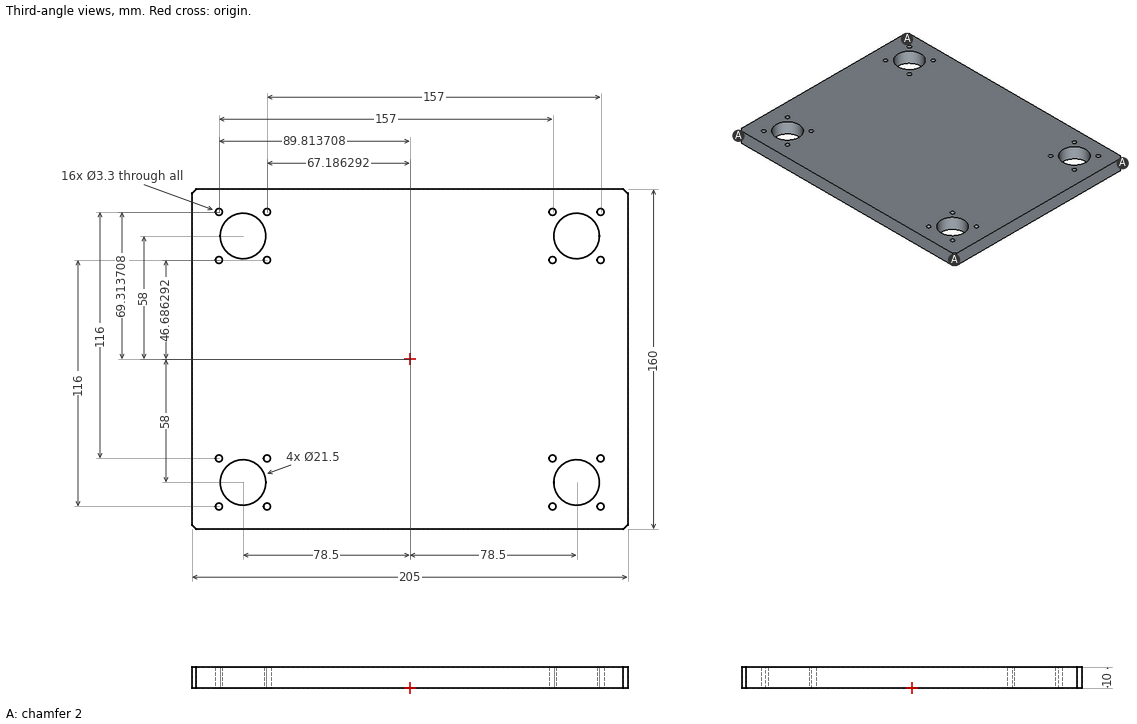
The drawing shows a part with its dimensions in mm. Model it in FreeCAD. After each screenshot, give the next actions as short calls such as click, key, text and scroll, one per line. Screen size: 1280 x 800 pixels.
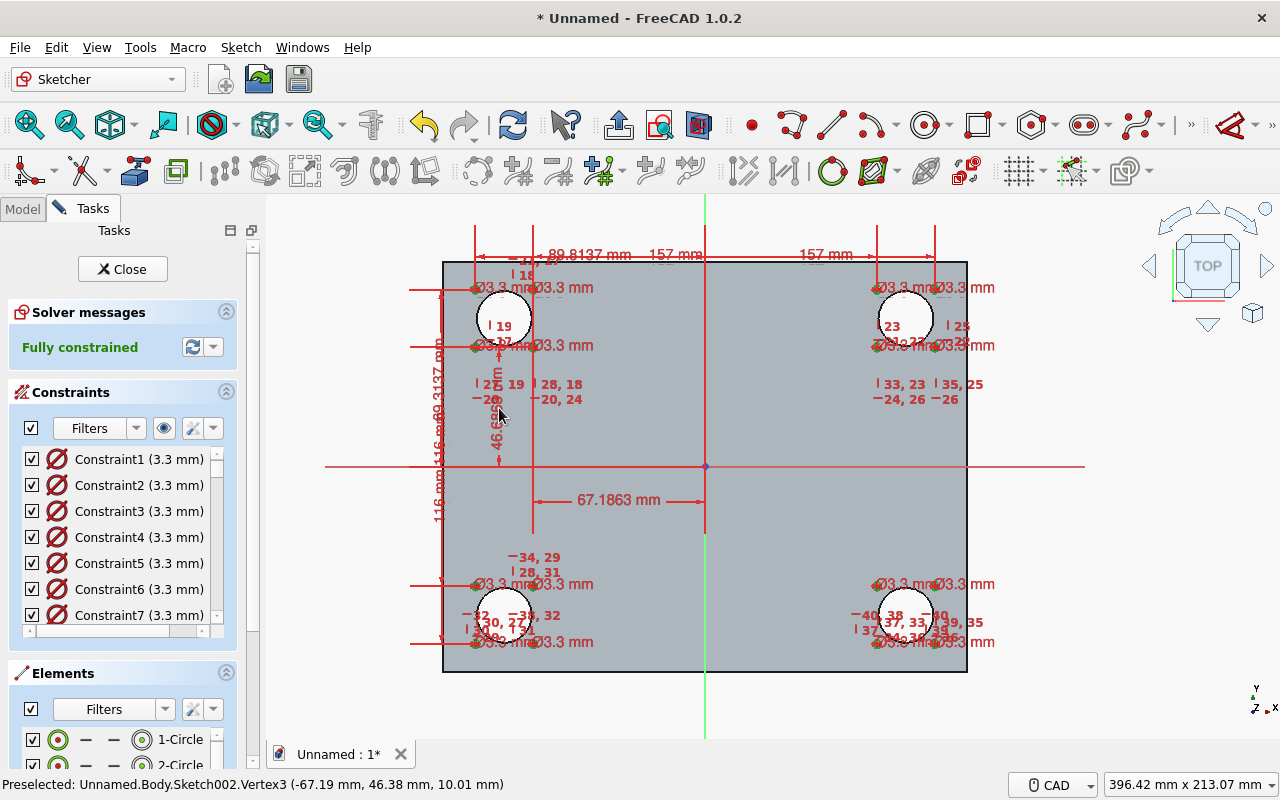
click(123, 269)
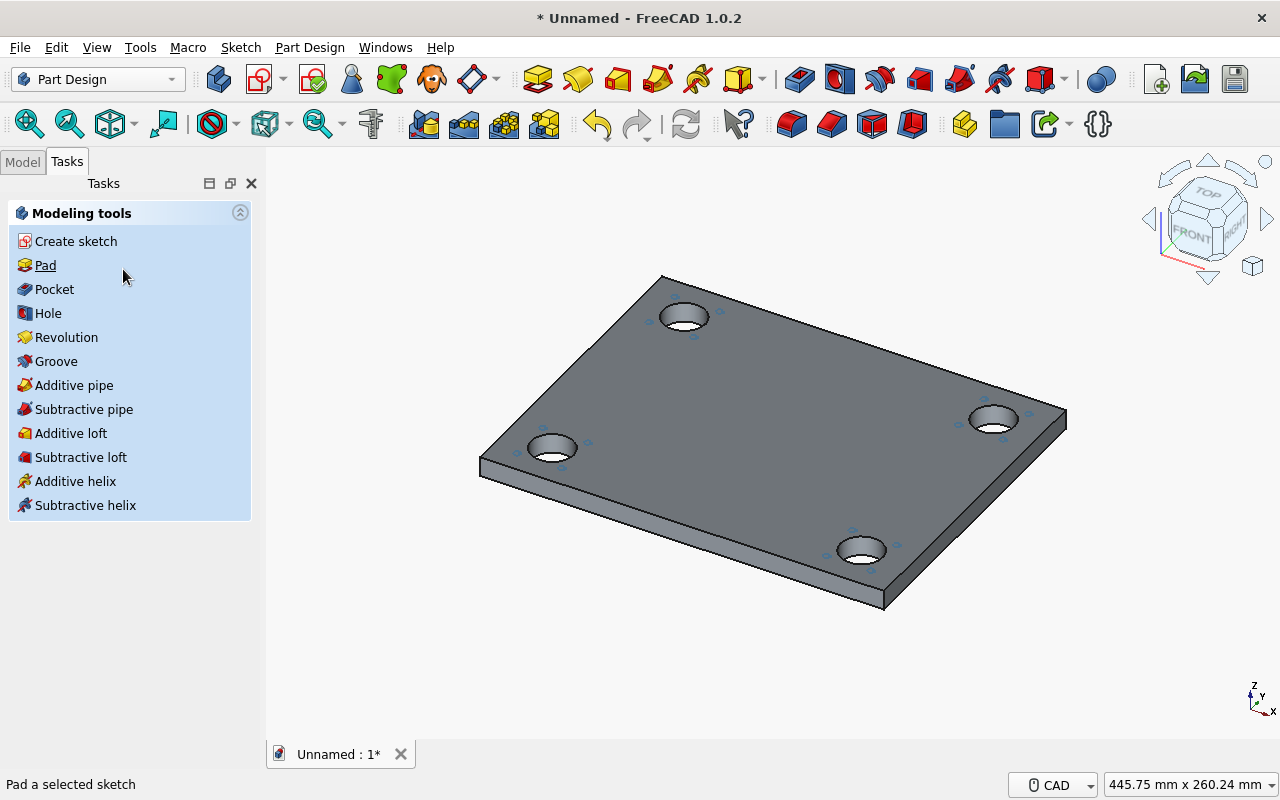
click(840, 80)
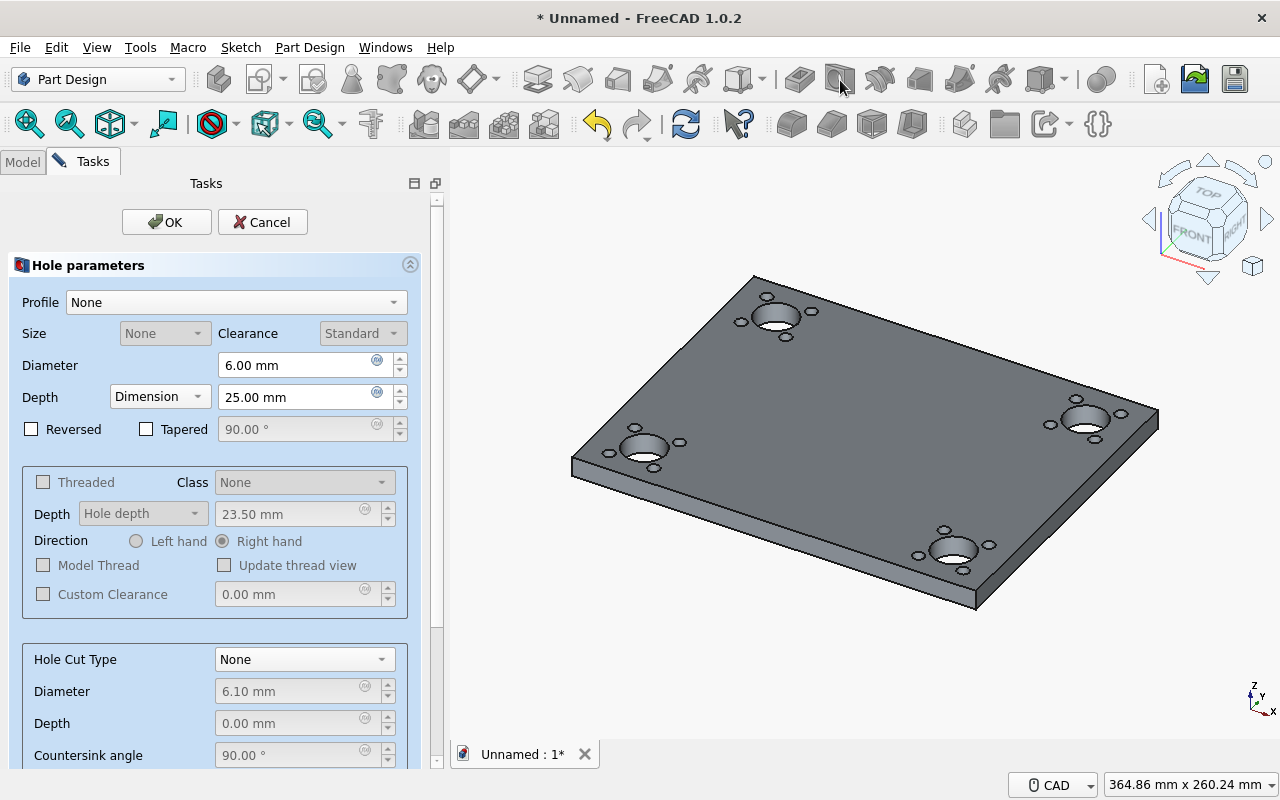
triple_click(305, 365)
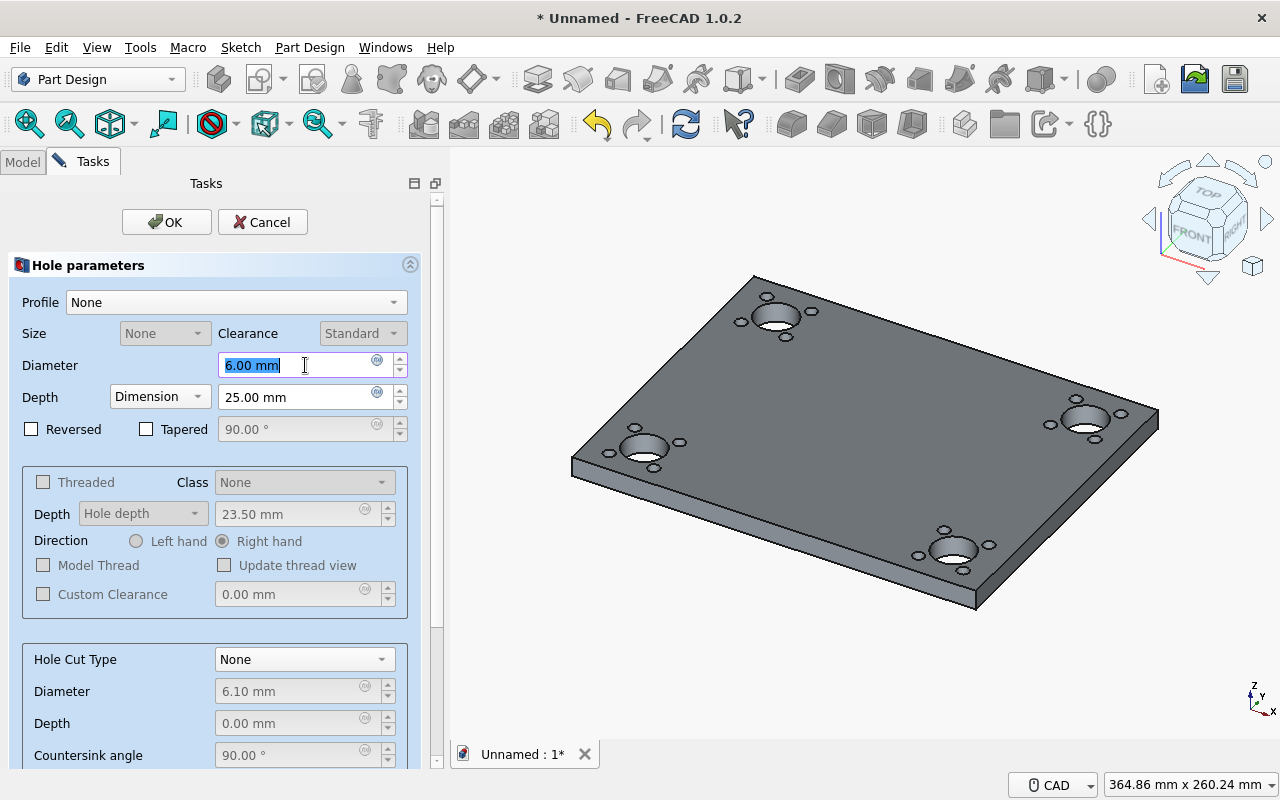
text(3.3)
key(Tab)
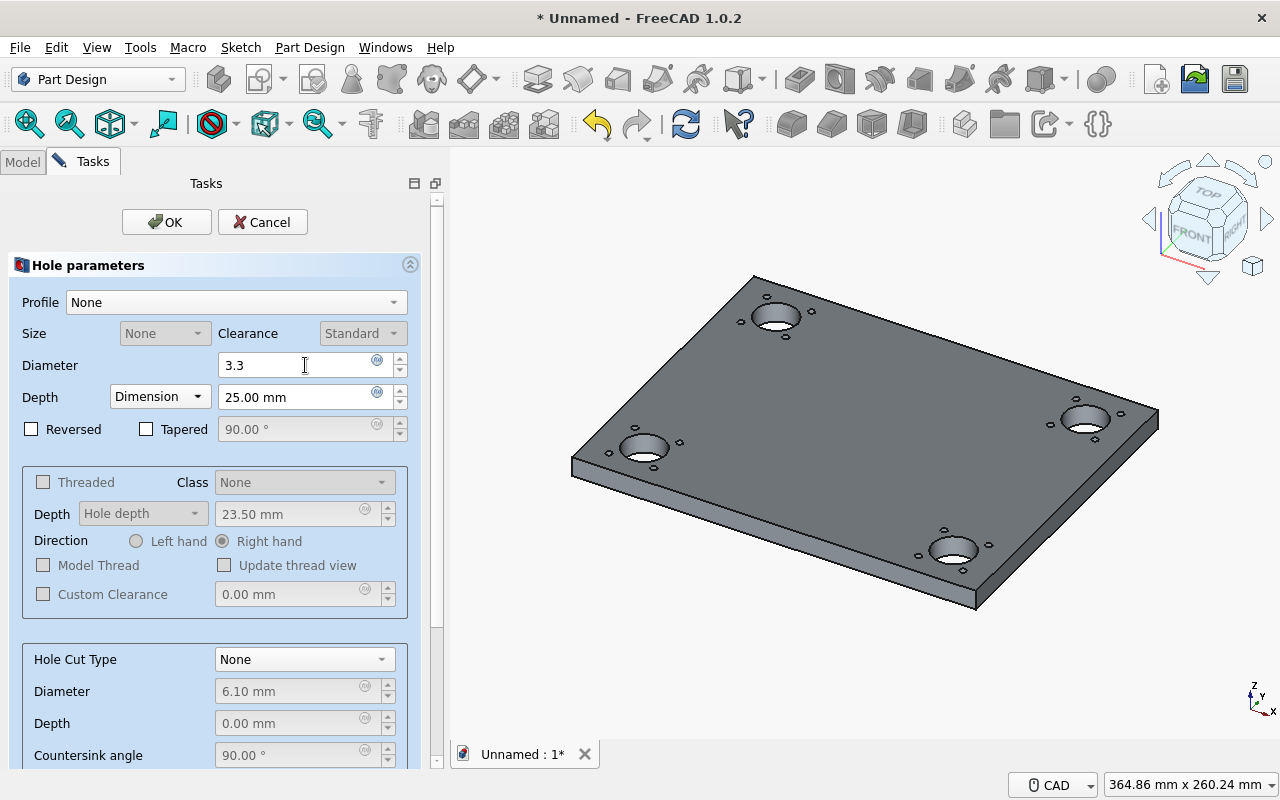
click(161, 396)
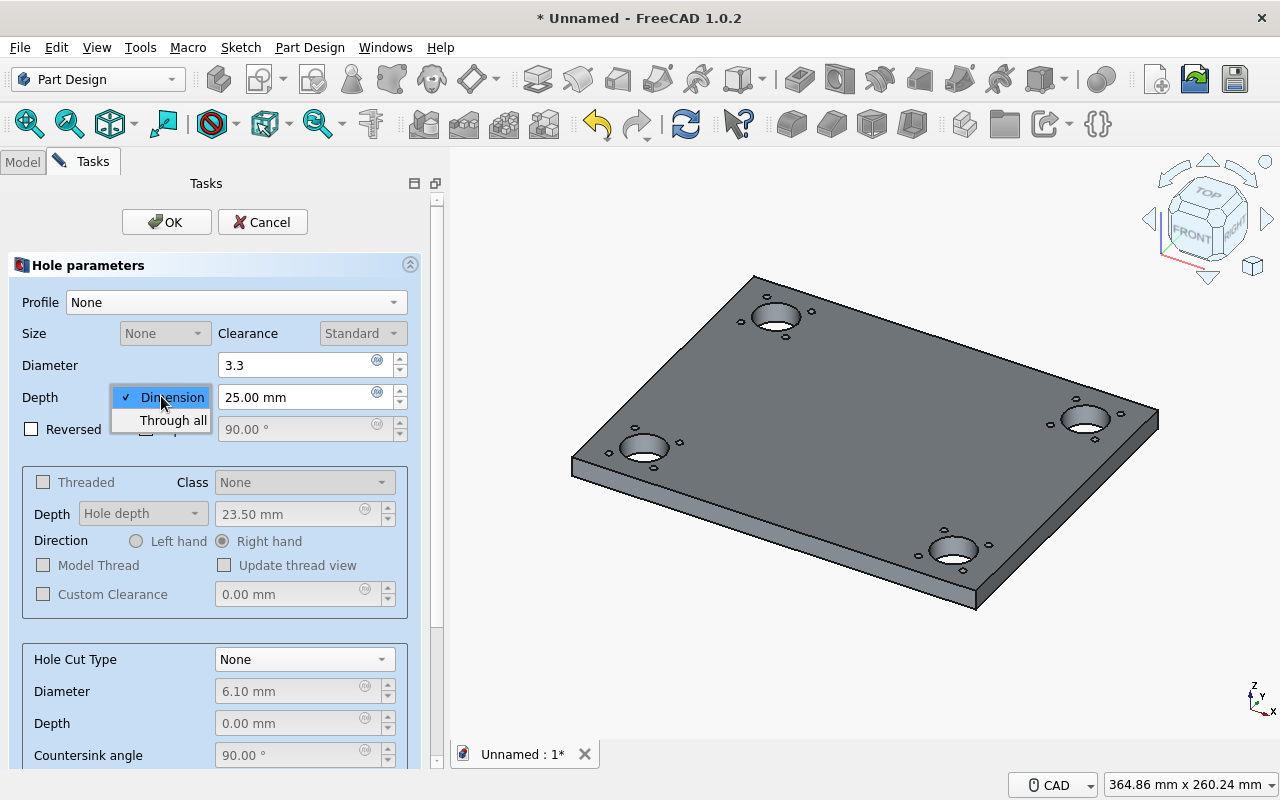
click(160, 420)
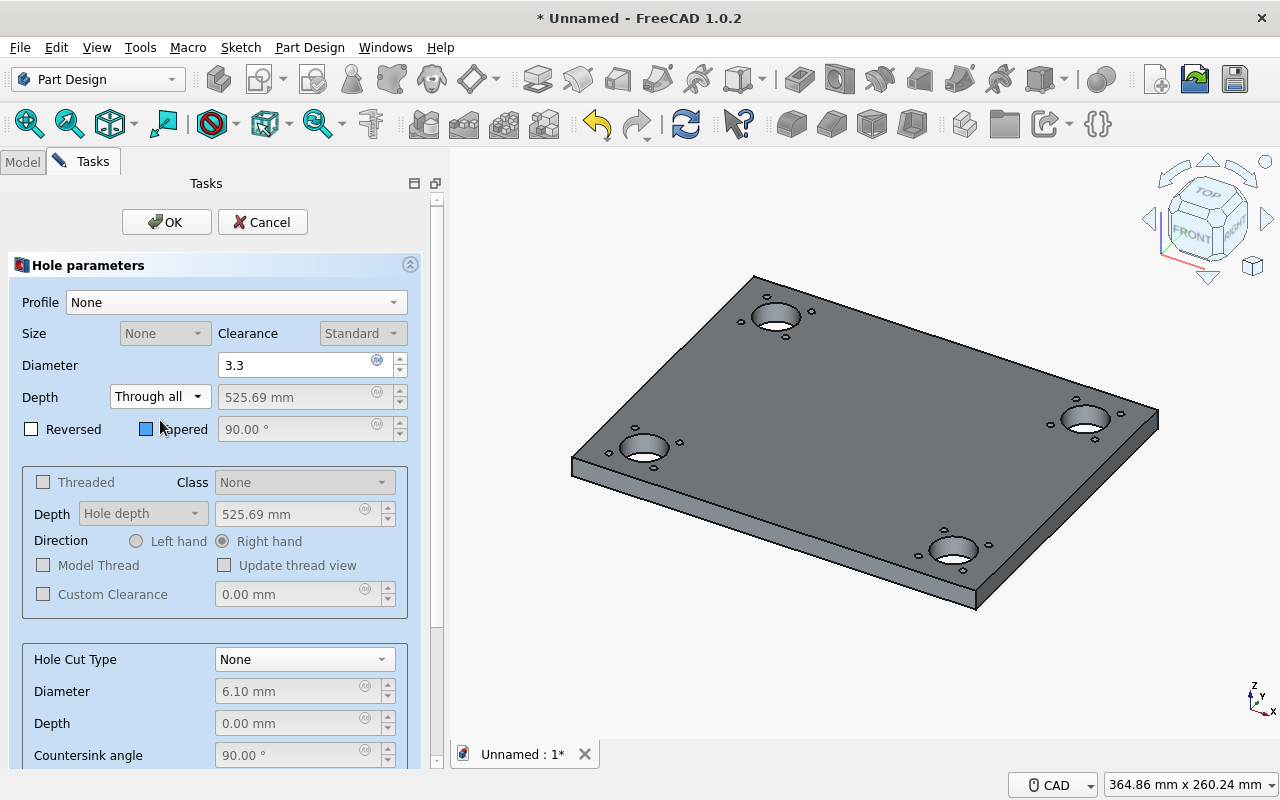
click(167, 222)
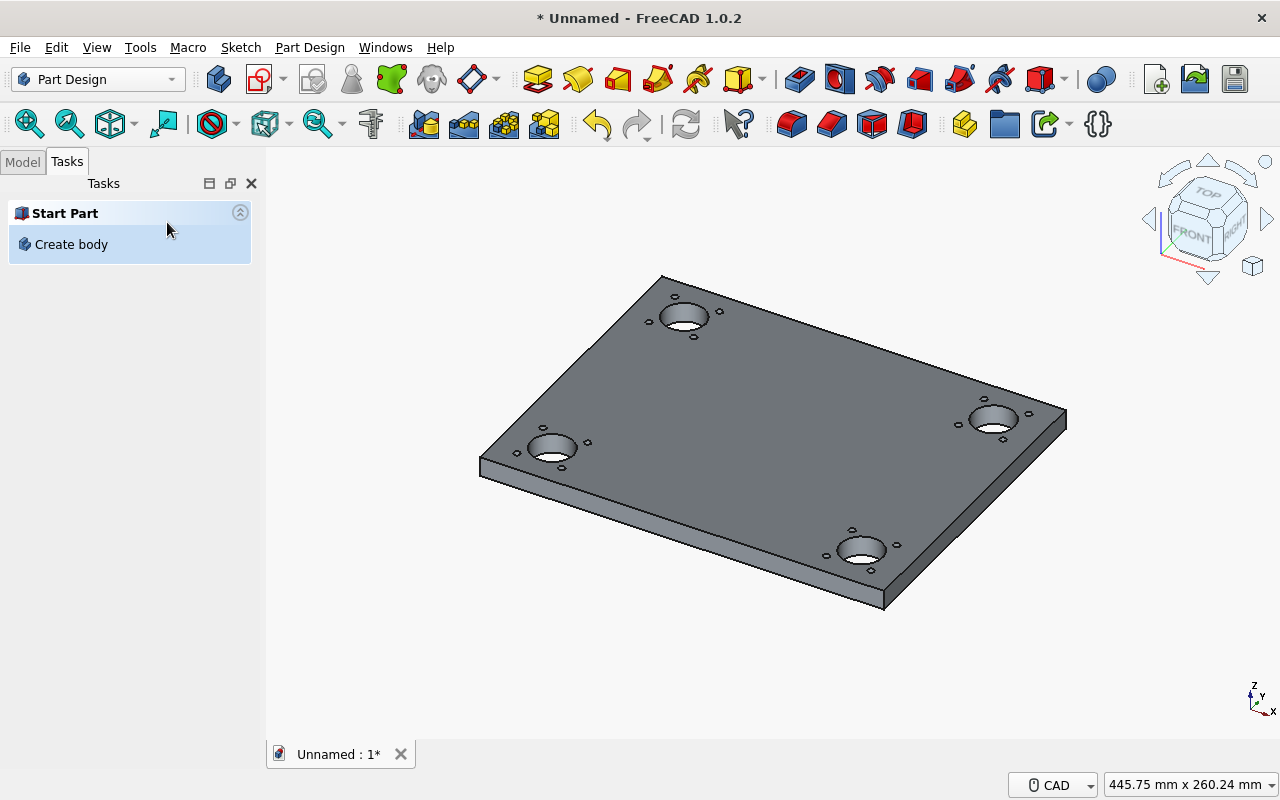
click(884, 599)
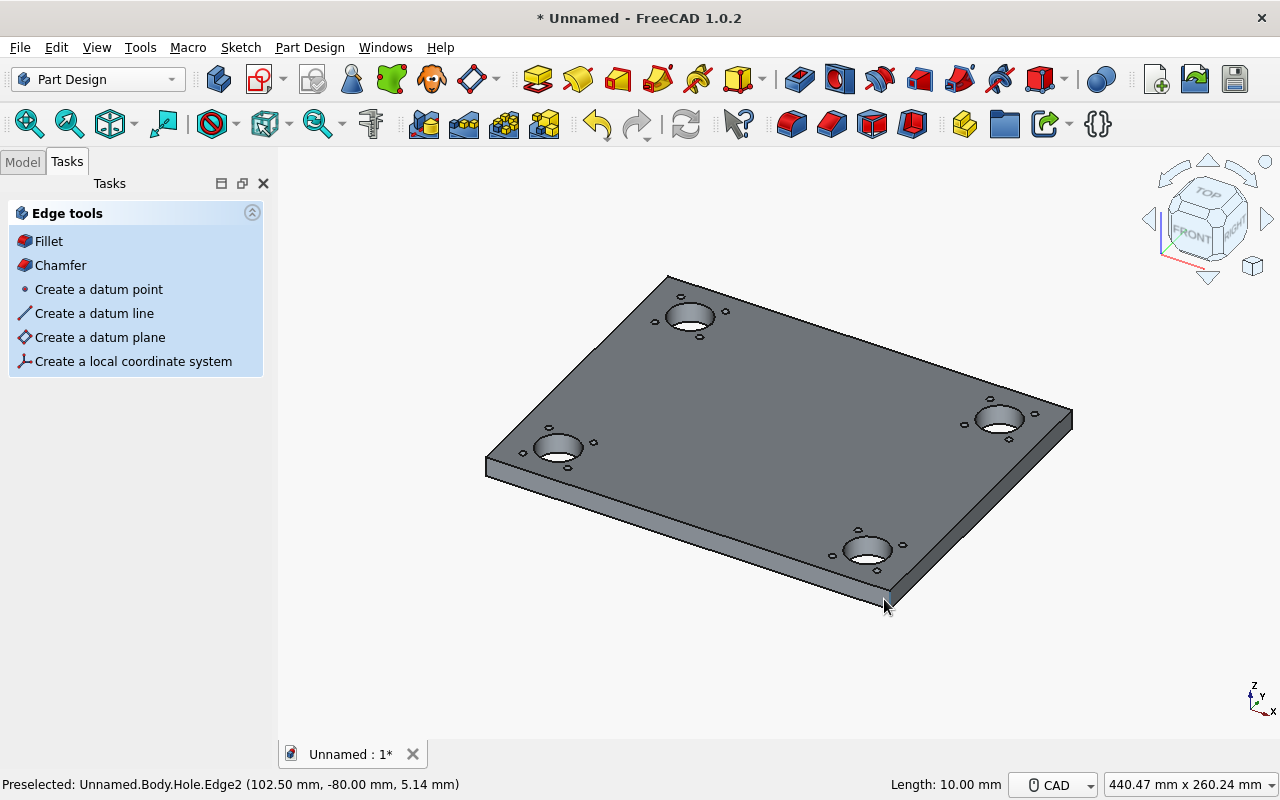
key(0)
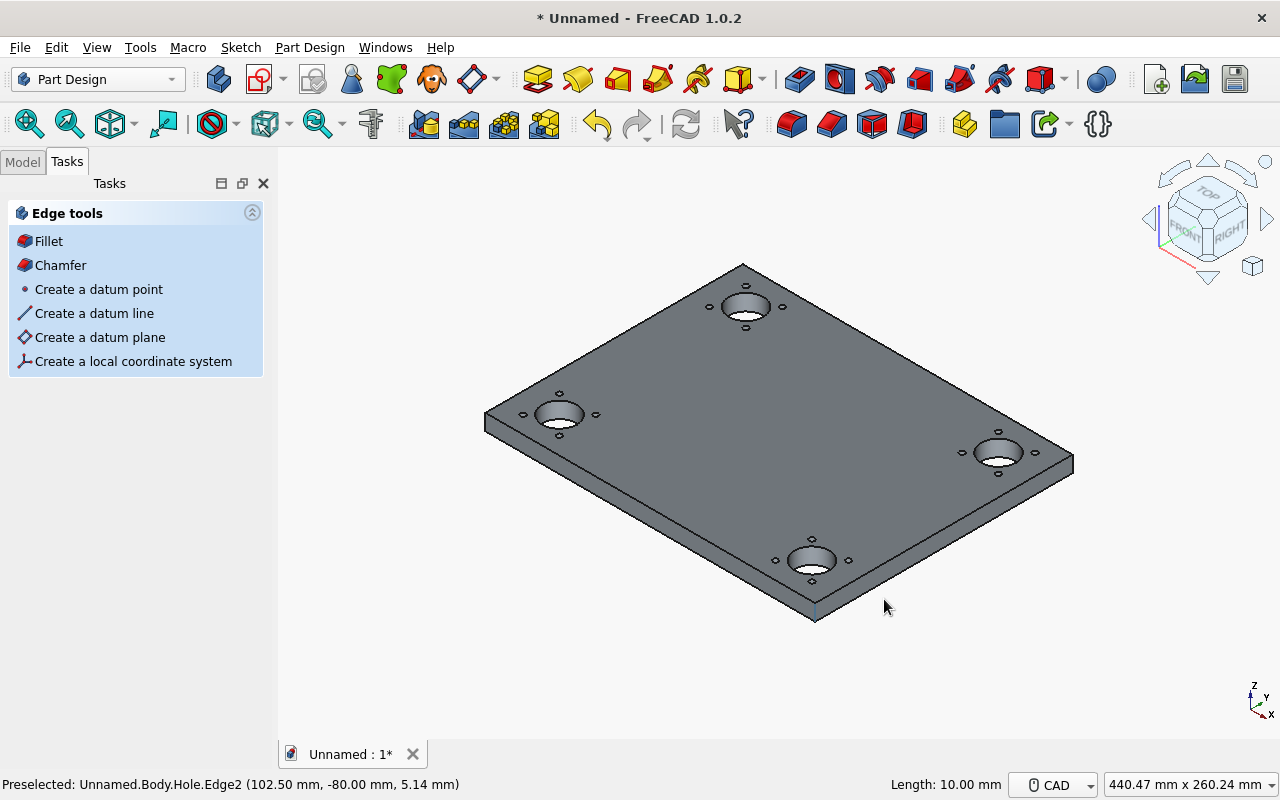
key(2)